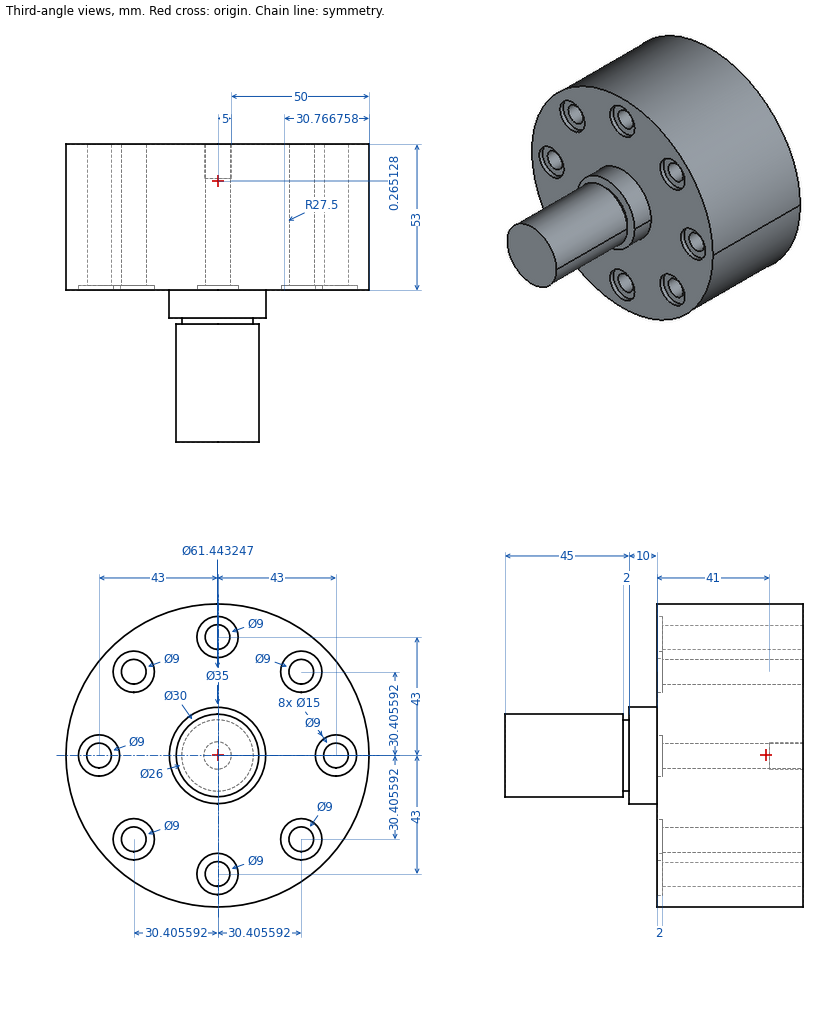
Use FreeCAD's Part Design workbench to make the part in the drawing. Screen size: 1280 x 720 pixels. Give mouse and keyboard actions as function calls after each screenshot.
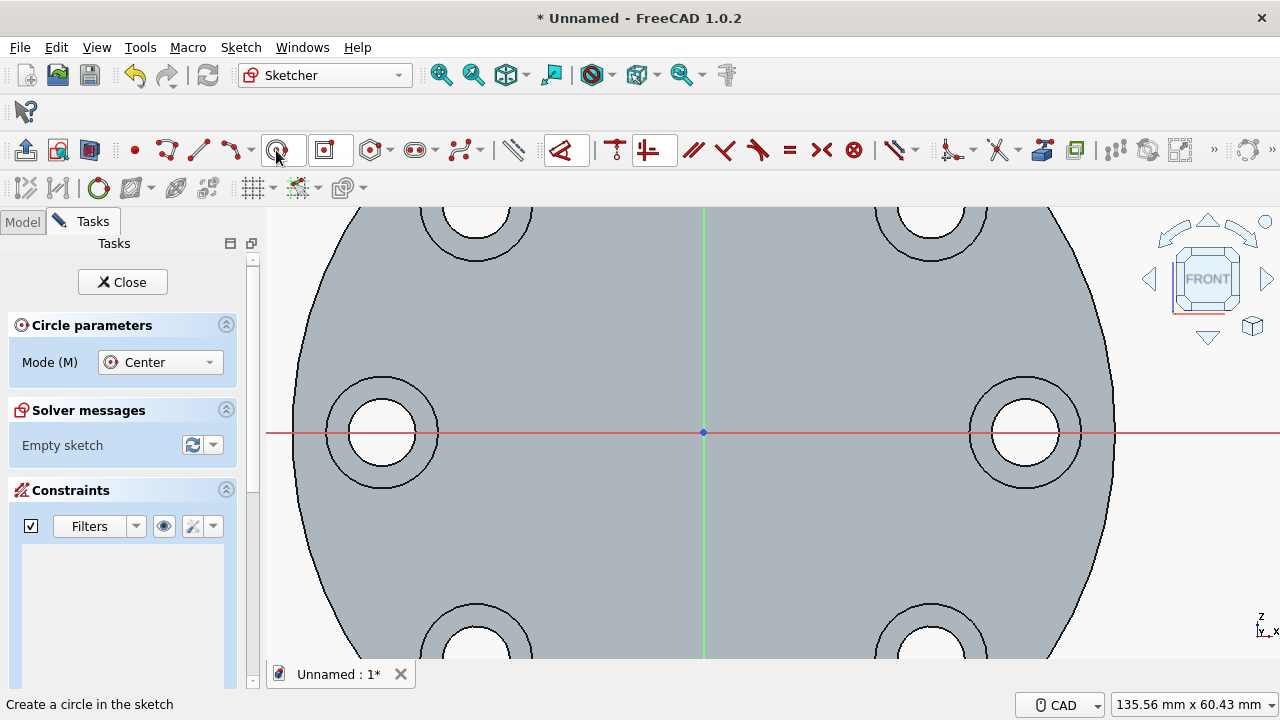
click(704, 433)
move(796, 340)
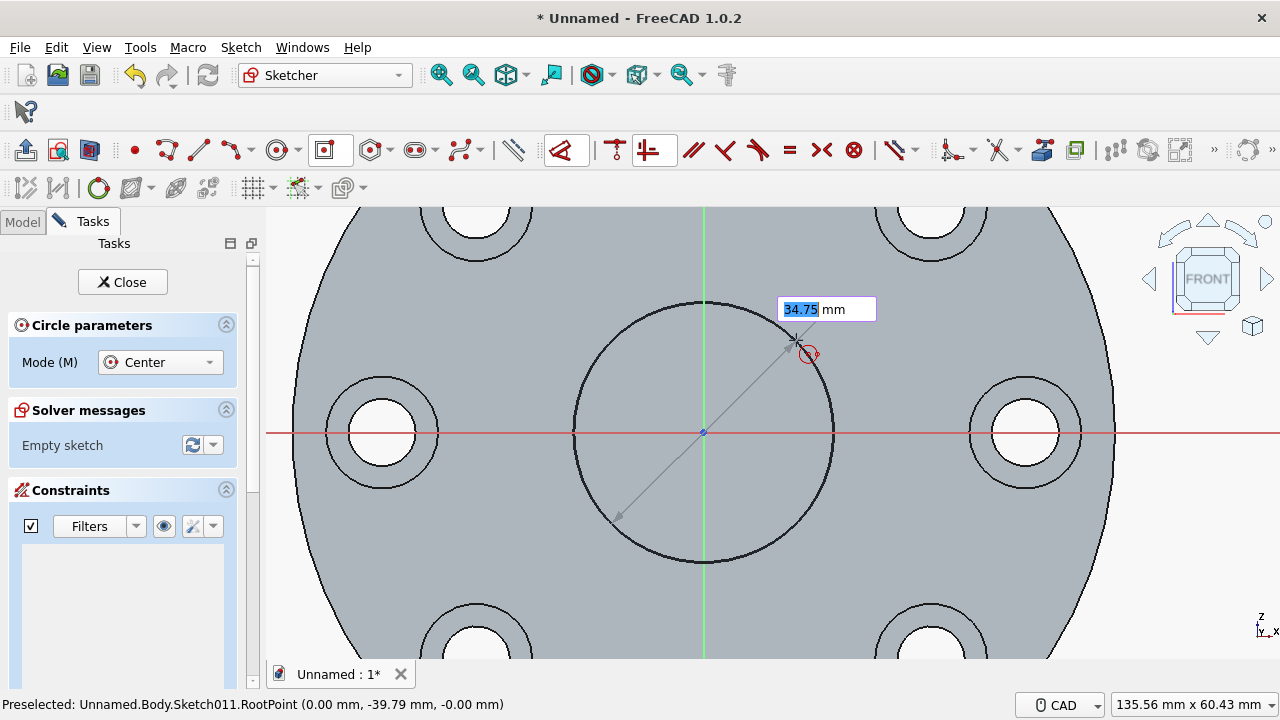
text(35)
key(Return)
key(Escape)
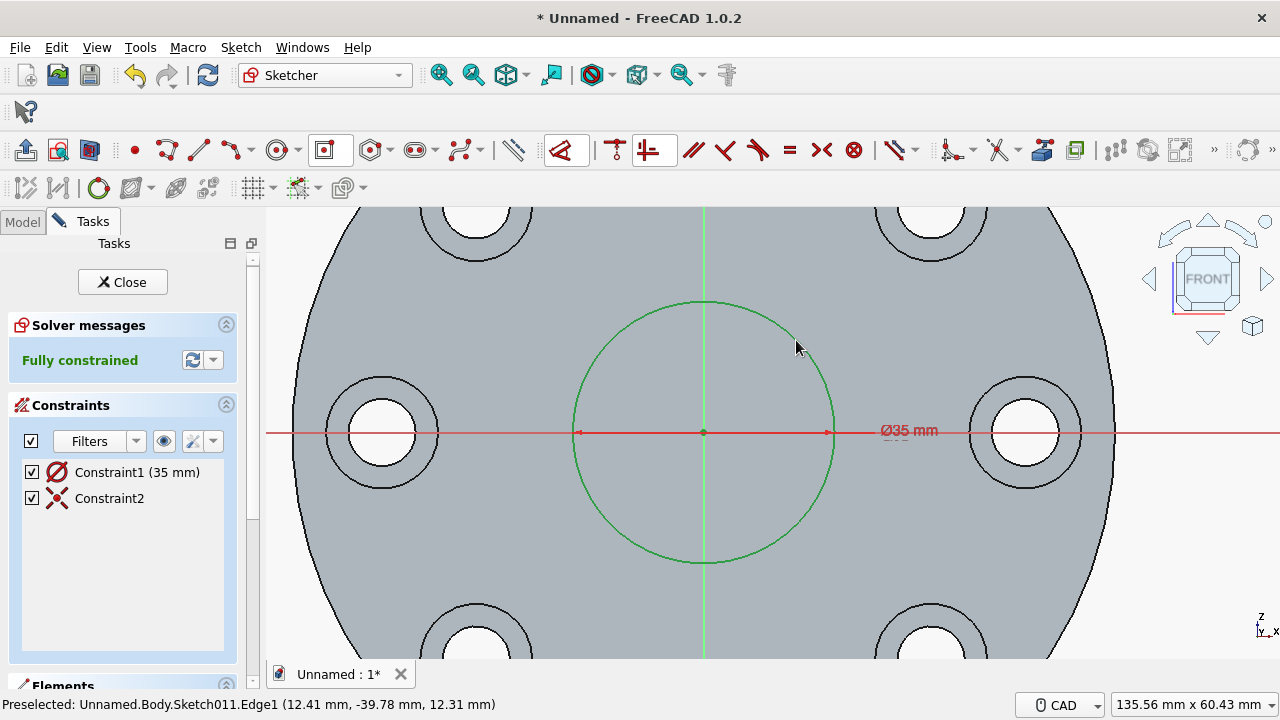
click(123, 282)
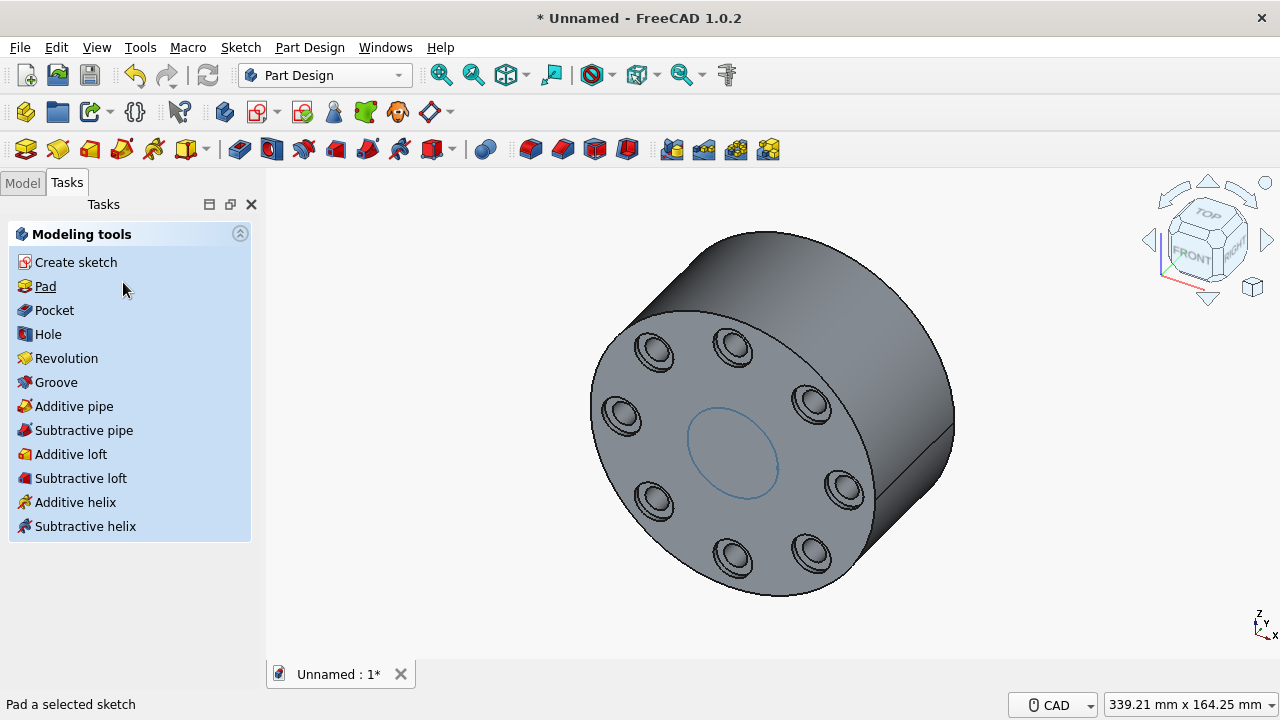
click(26, 150)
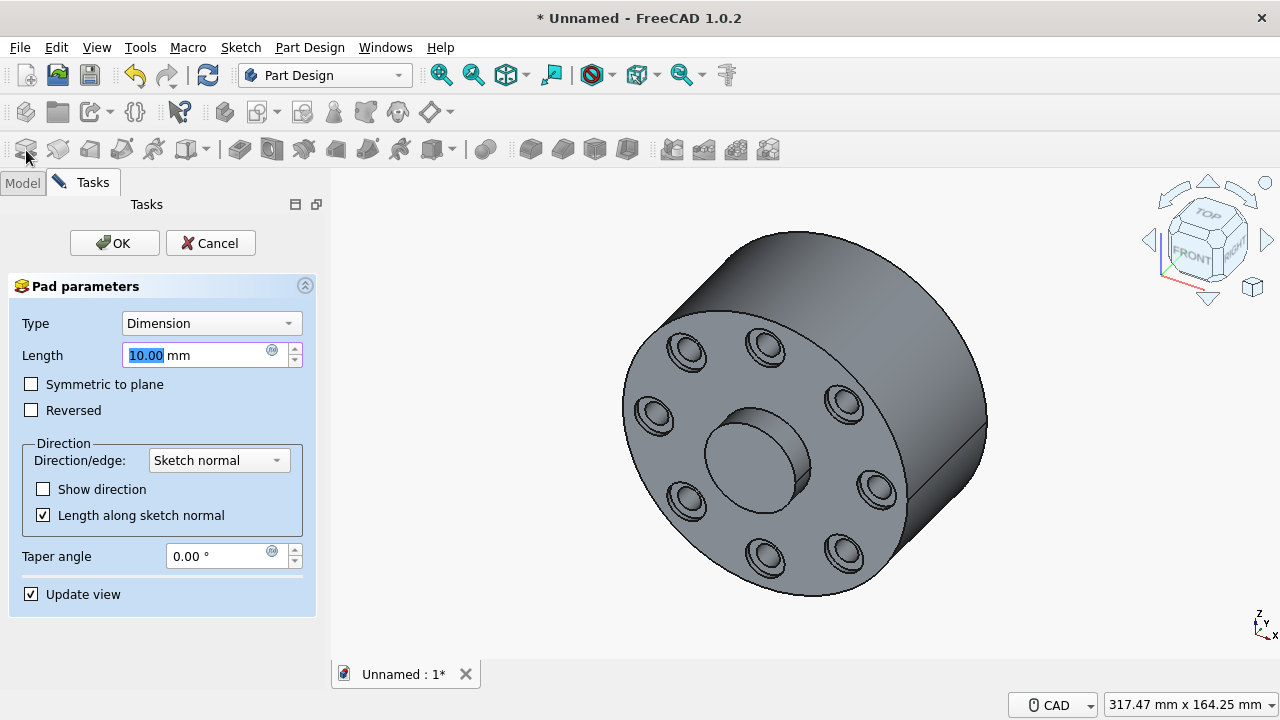
text(10)
key(Tab)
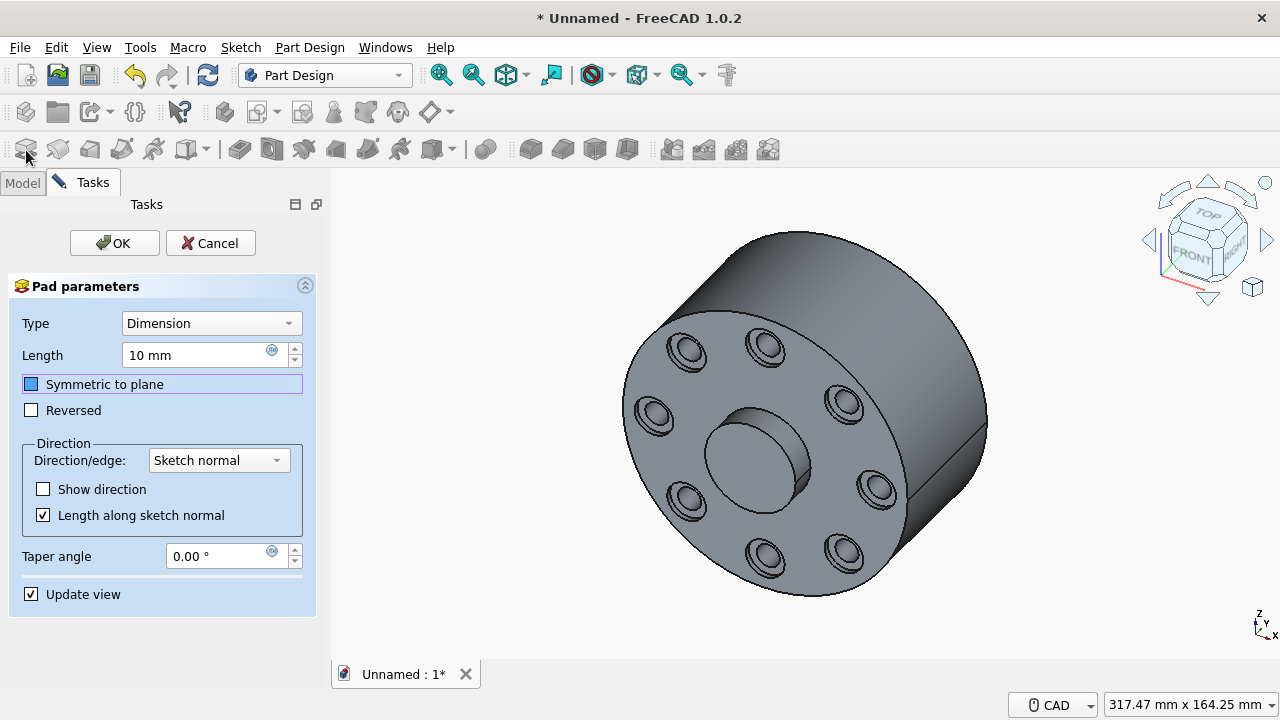
click(115, 243)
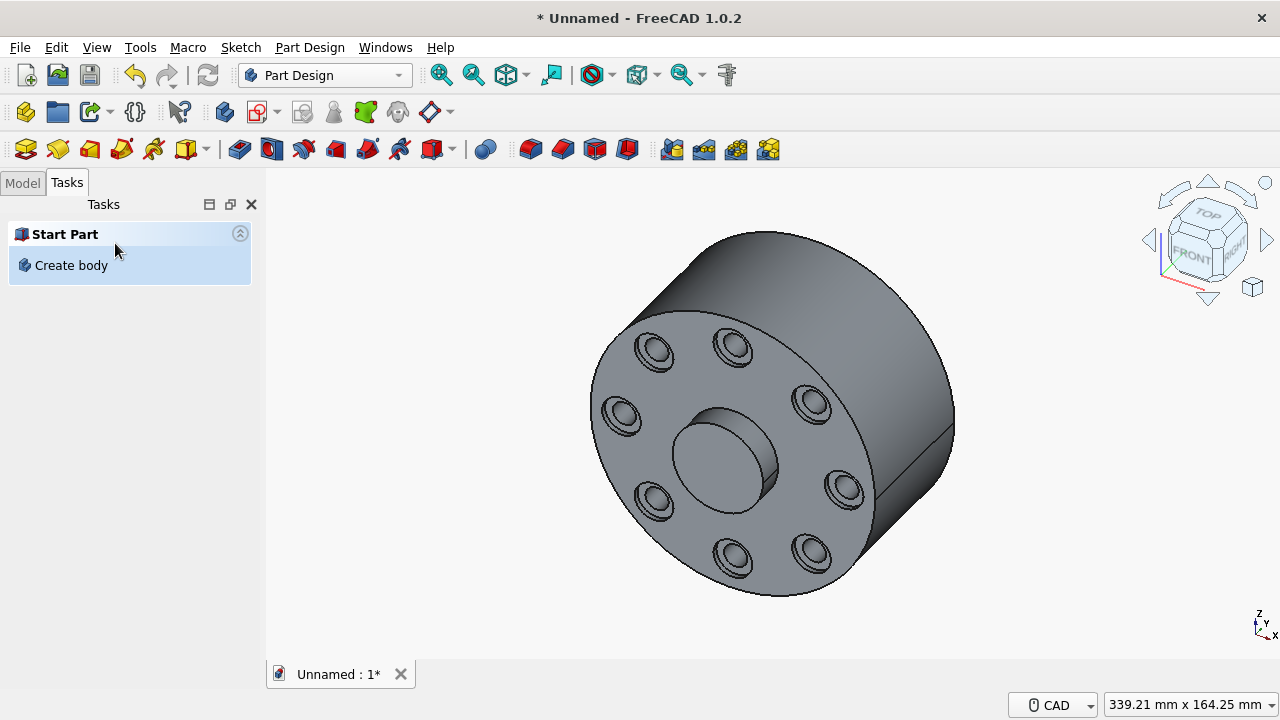
click(718, 467)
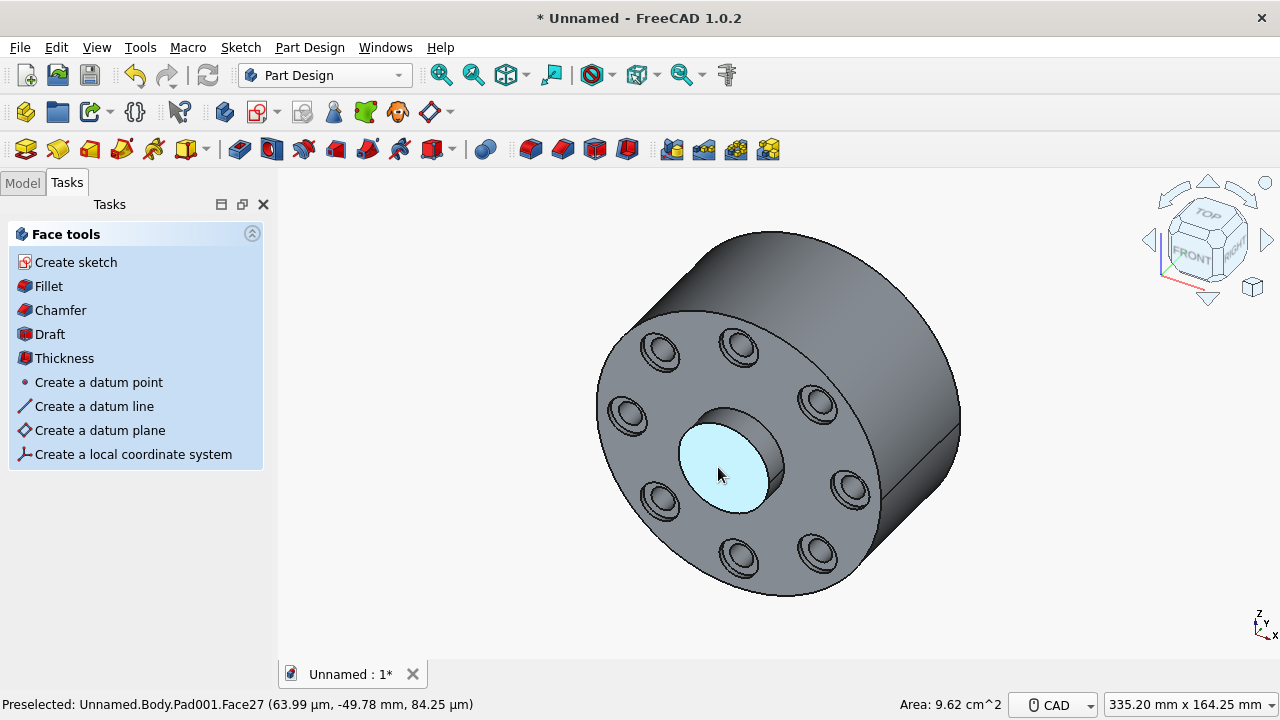
click(258, 112)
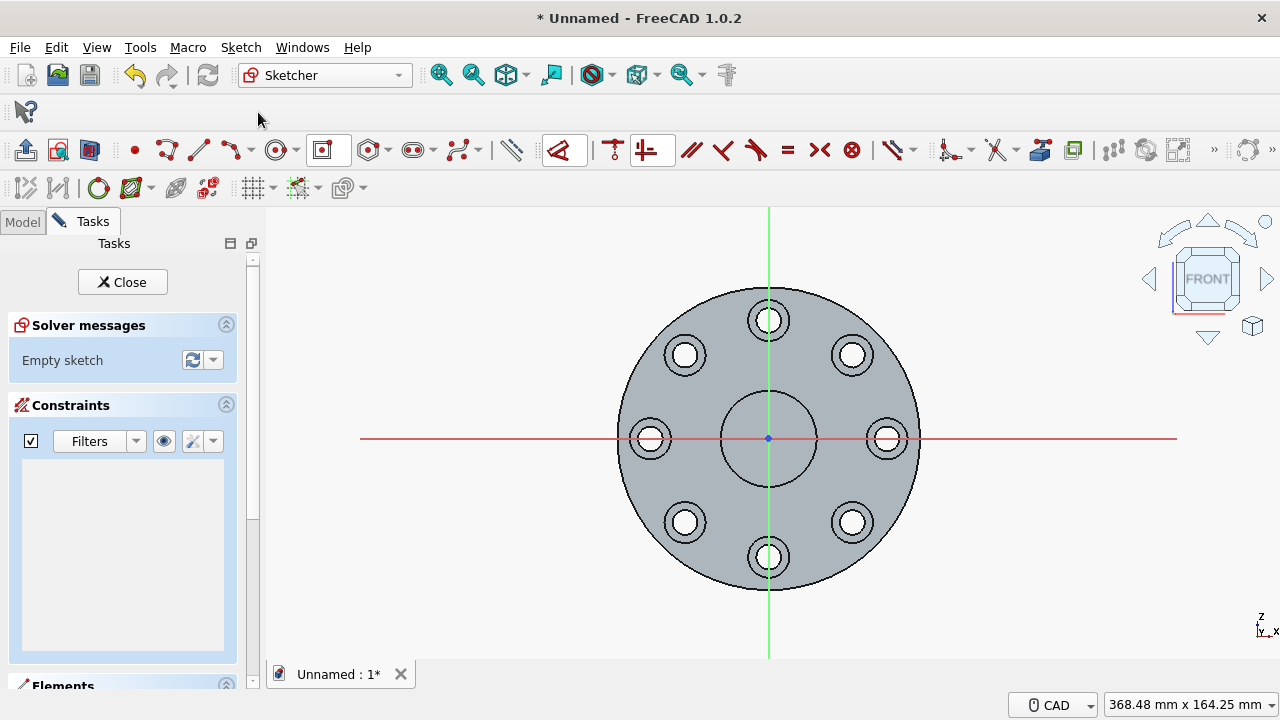
scroll(796, 441, up, 6)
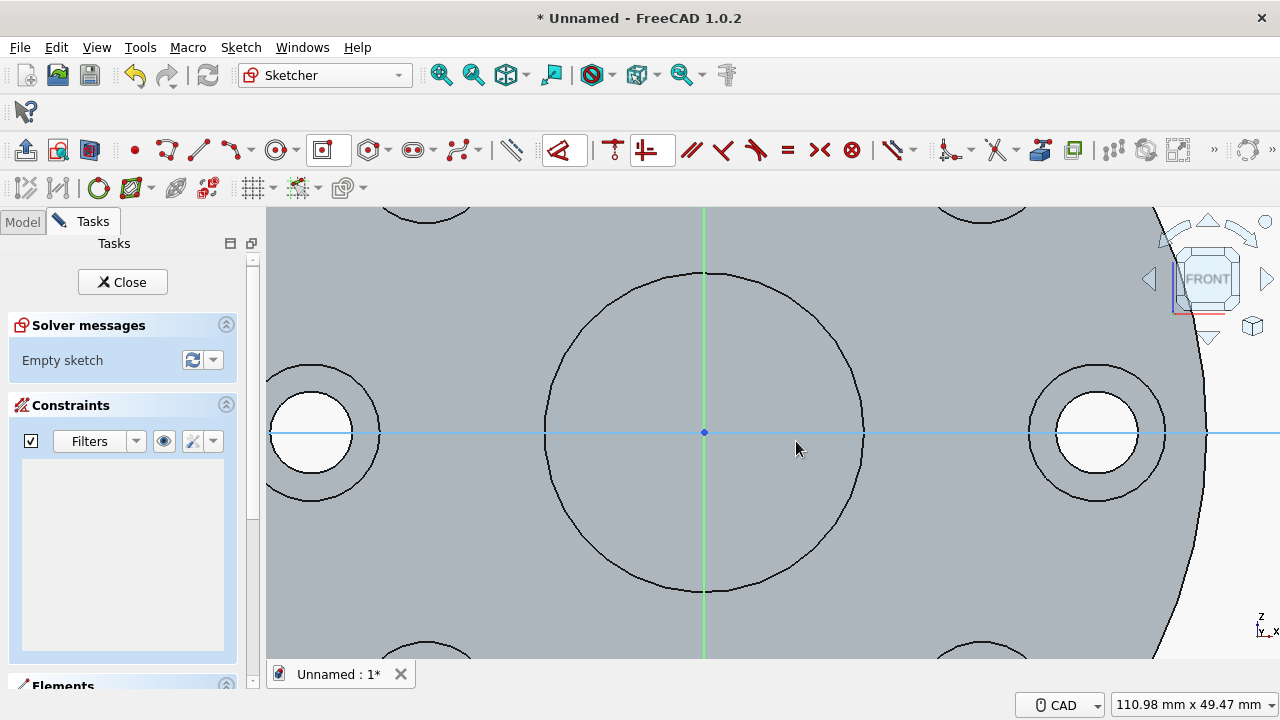
key(g)
key(c)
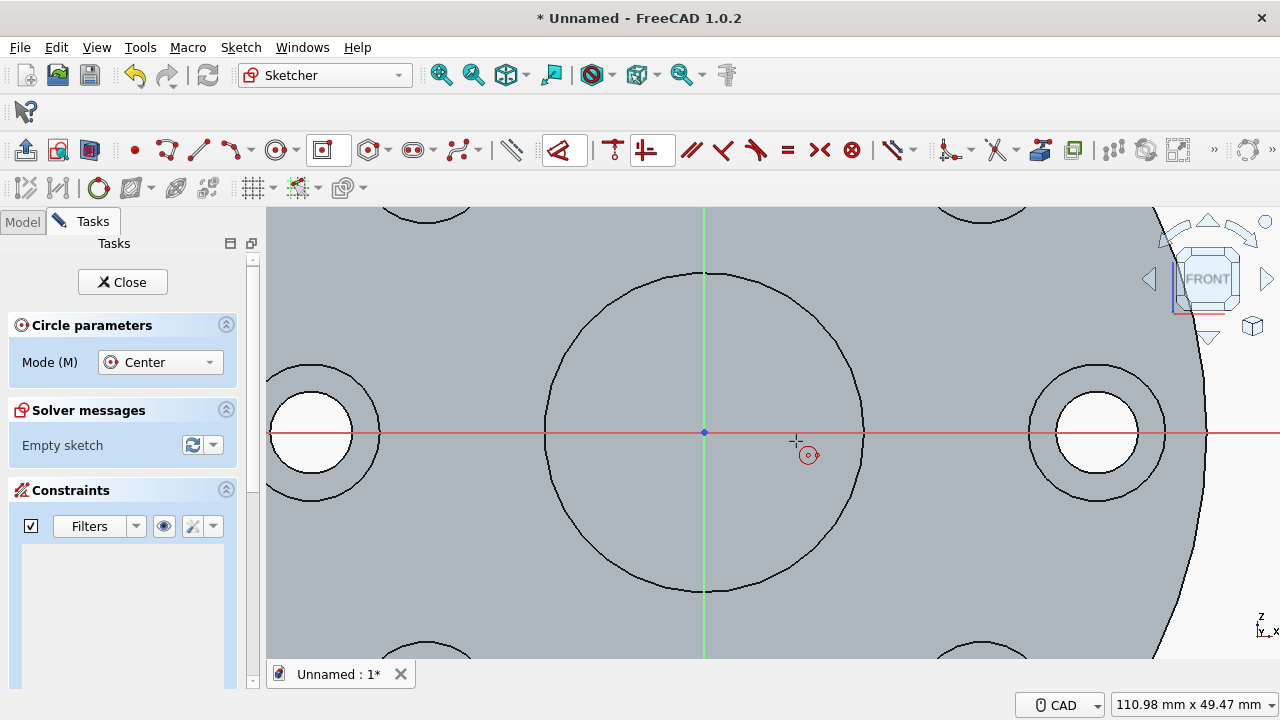
click(704, 433)
move(801, 336)